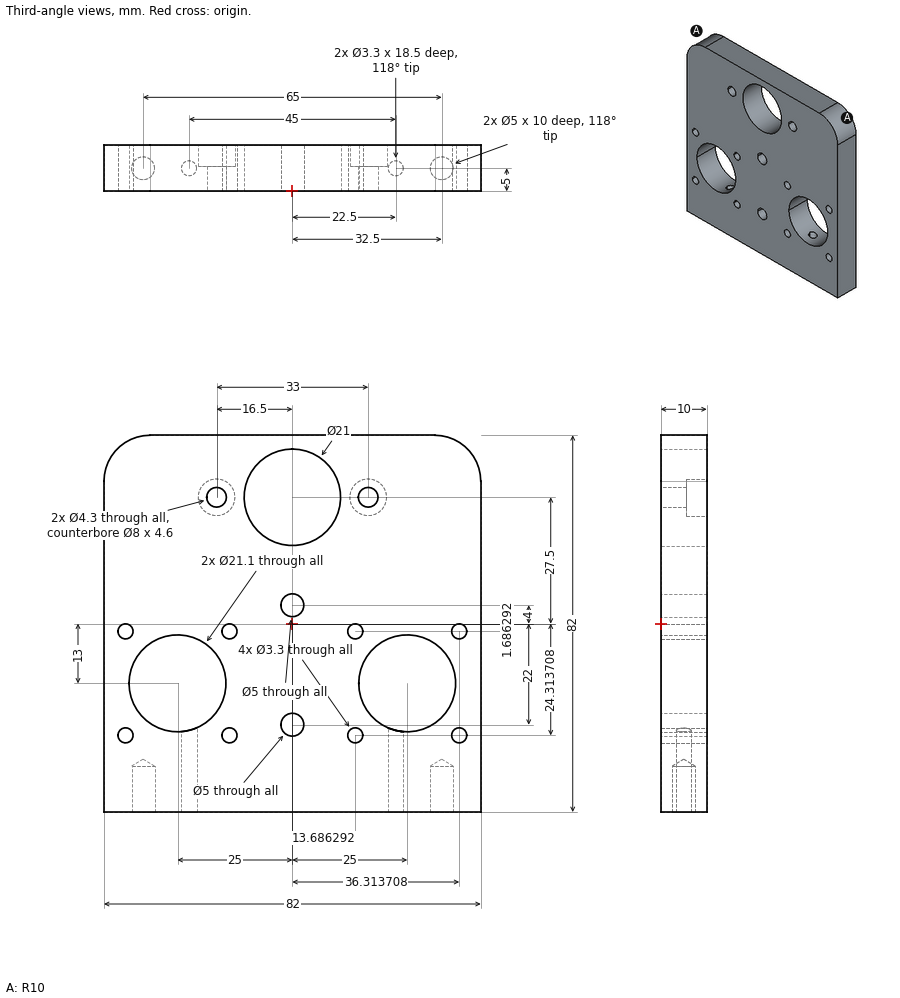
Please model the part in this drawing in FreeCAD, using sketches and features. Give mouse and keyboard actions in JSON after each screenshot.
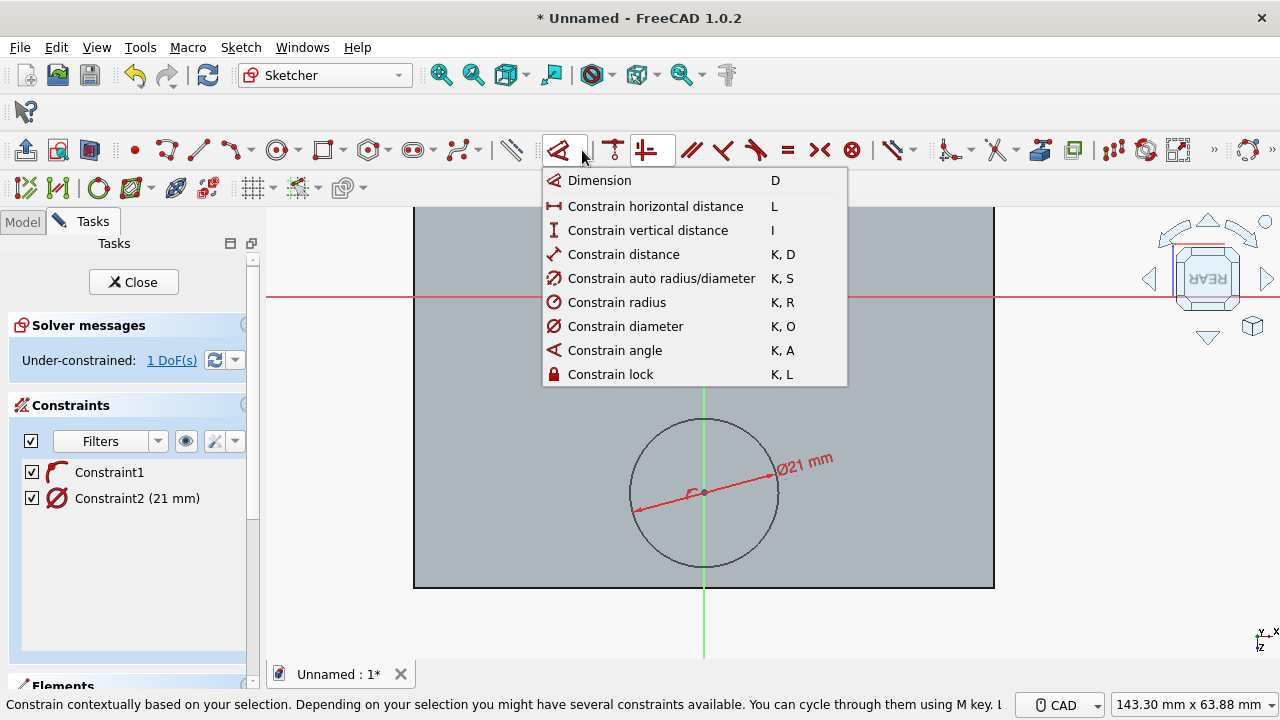
{"action": "left_click", "coordinate": [695, 230]}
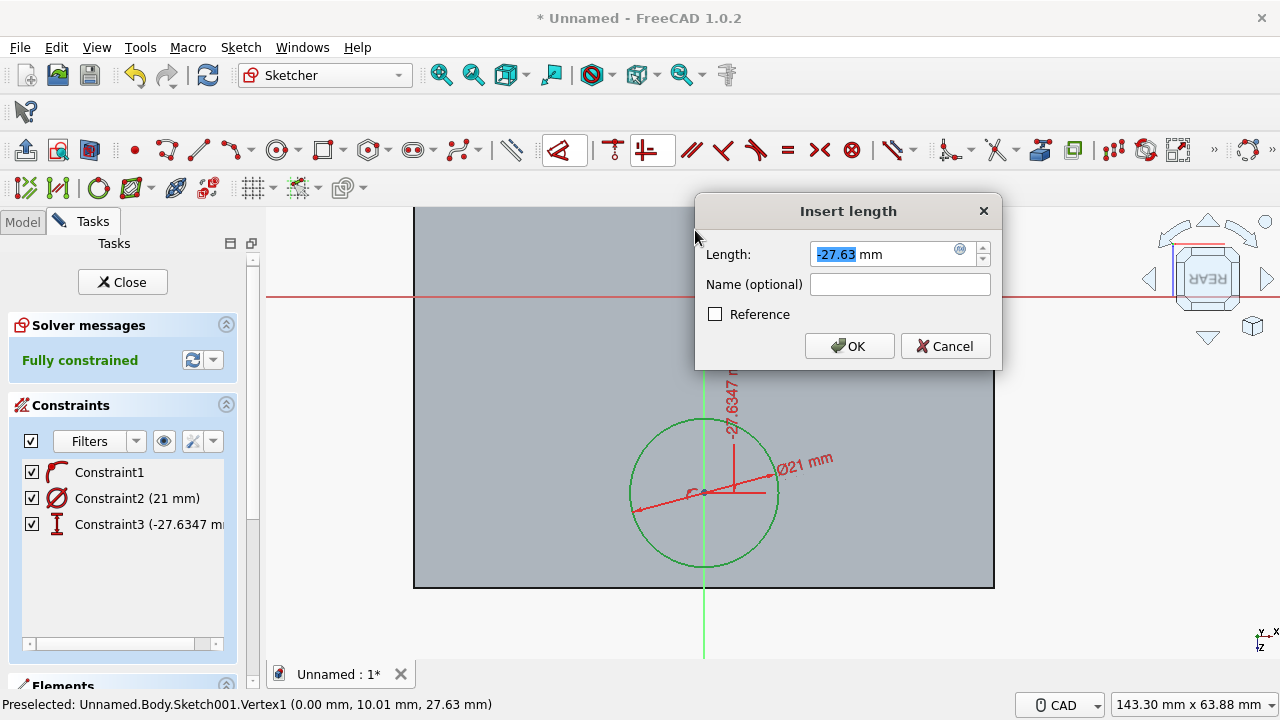
{"action": "type", "text": "-27.5"}
{"action": "key", "text": "Return"}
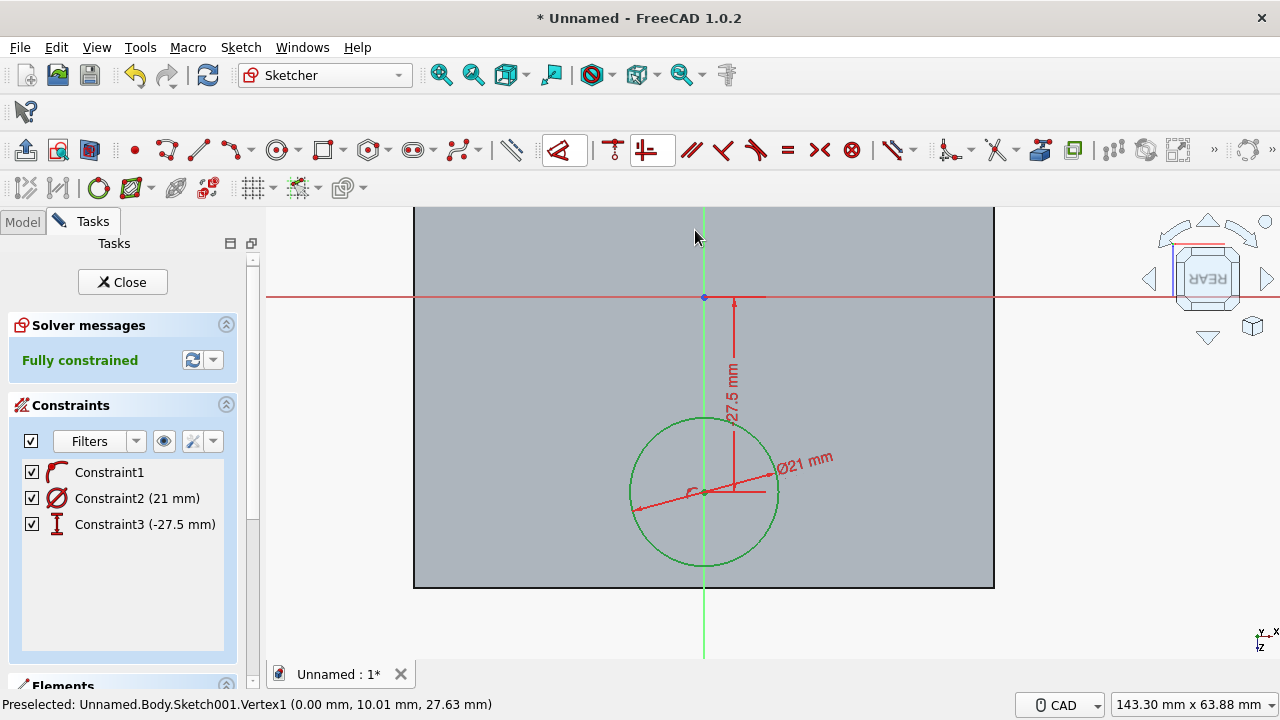
{"action": "left_click", "coordinate": [123, 282]}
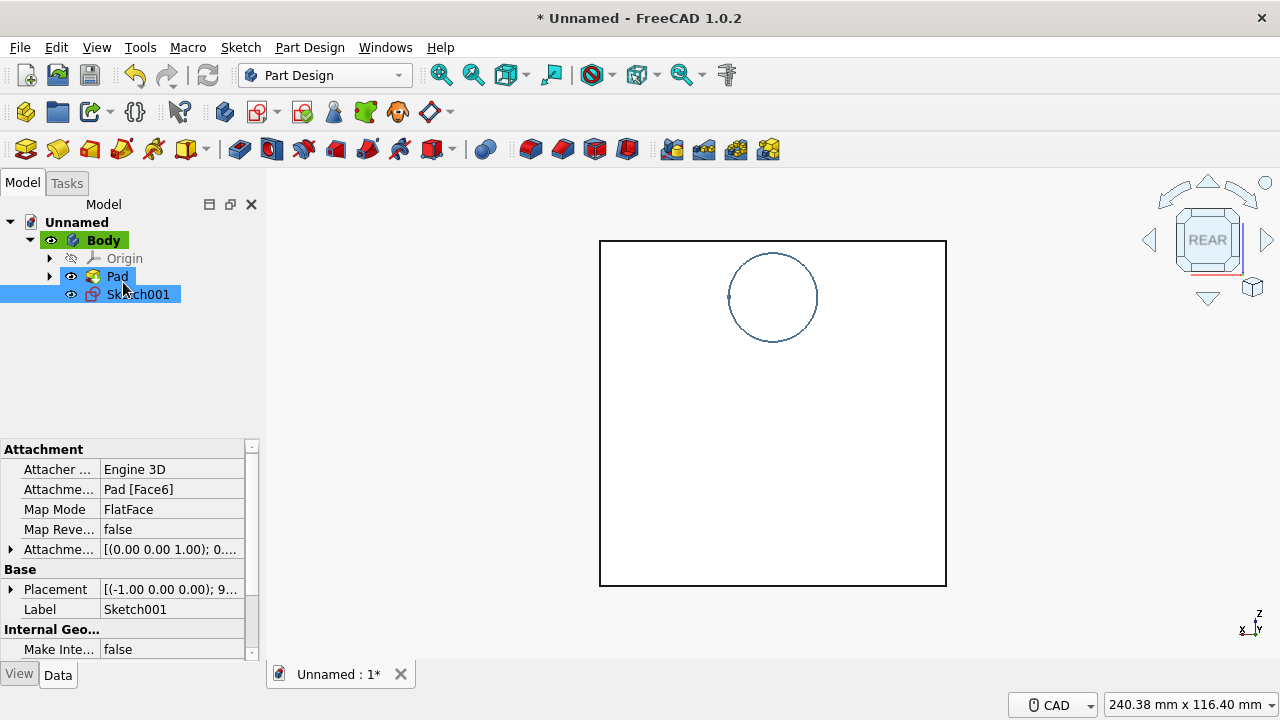
{"action": "left_click", "coordinate": [240, 150]}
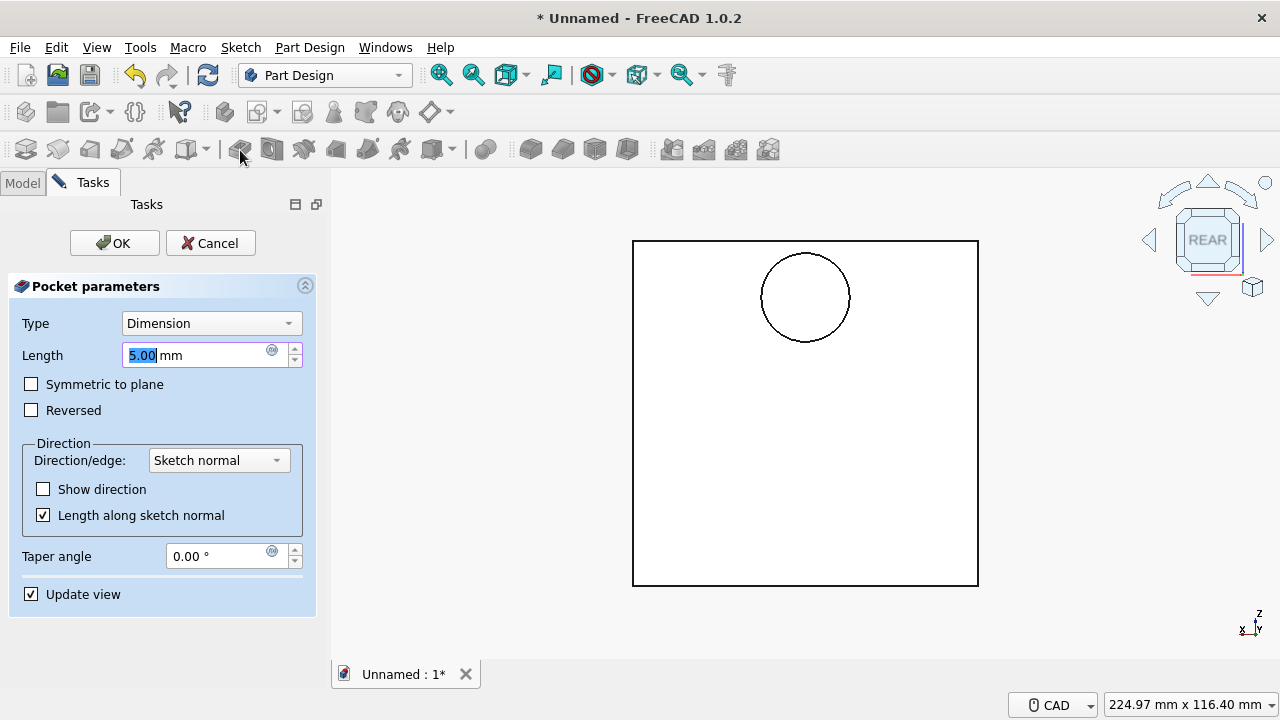
{"action": "left_click", "coordinate": [212, 324]}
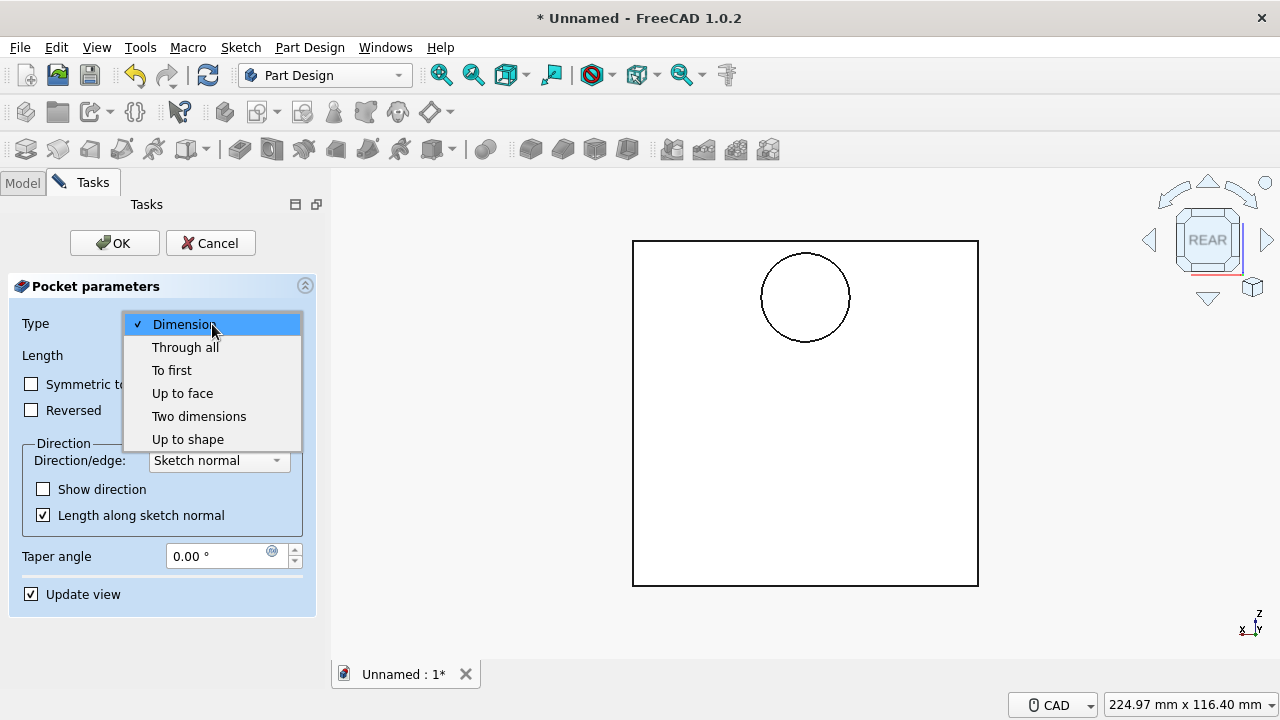
{"action": "left_click", "coordinate": [212, 348]}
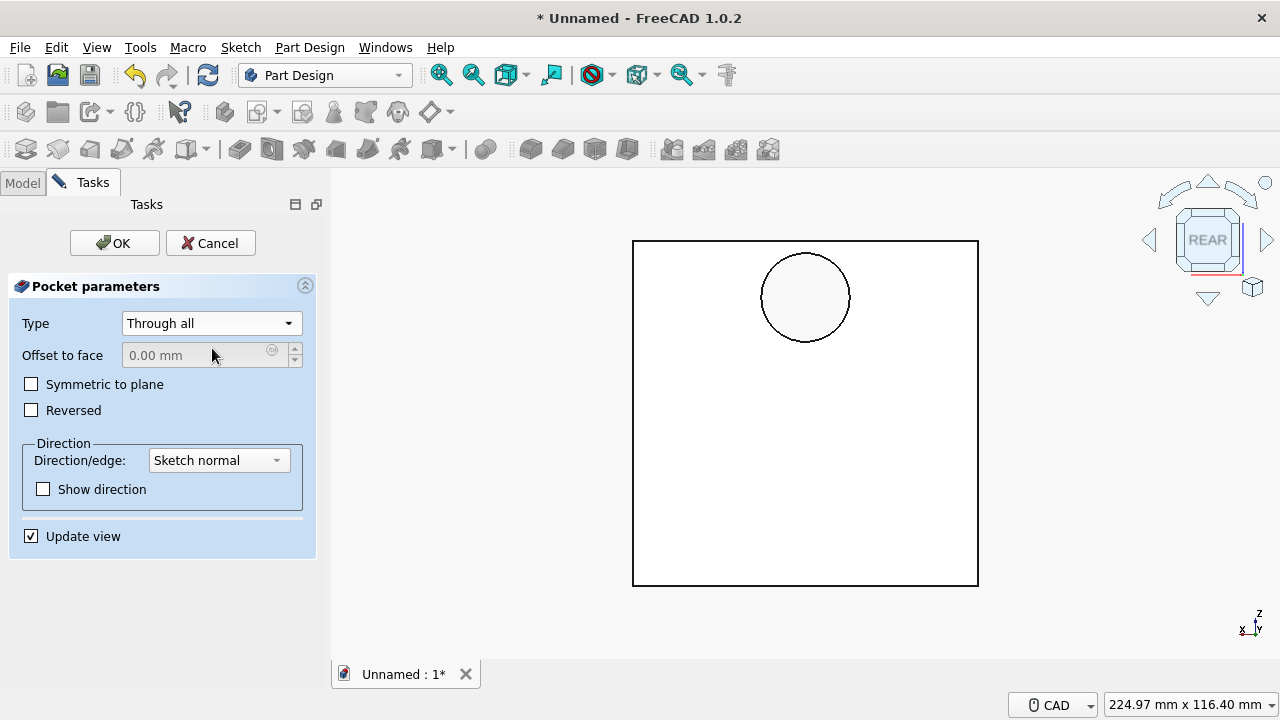
{"action": "left_click", "coordinate": [115, 243]}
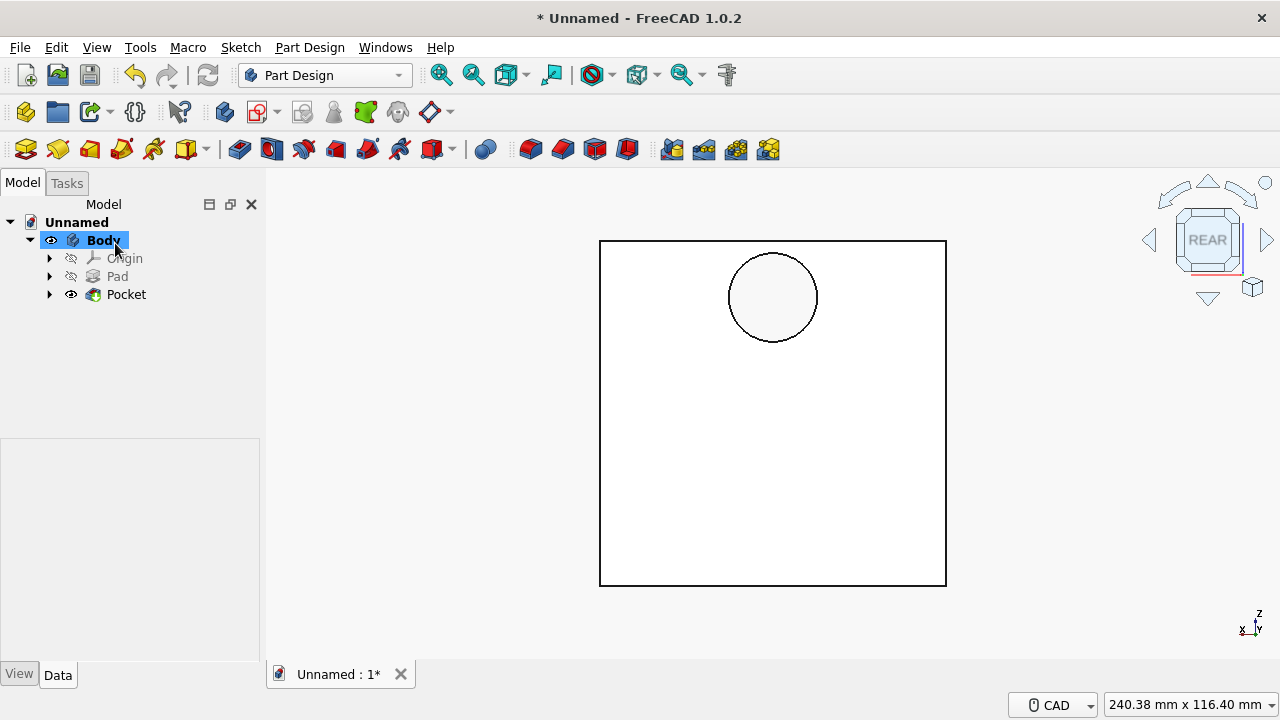
{"action": "key", "text": "0"}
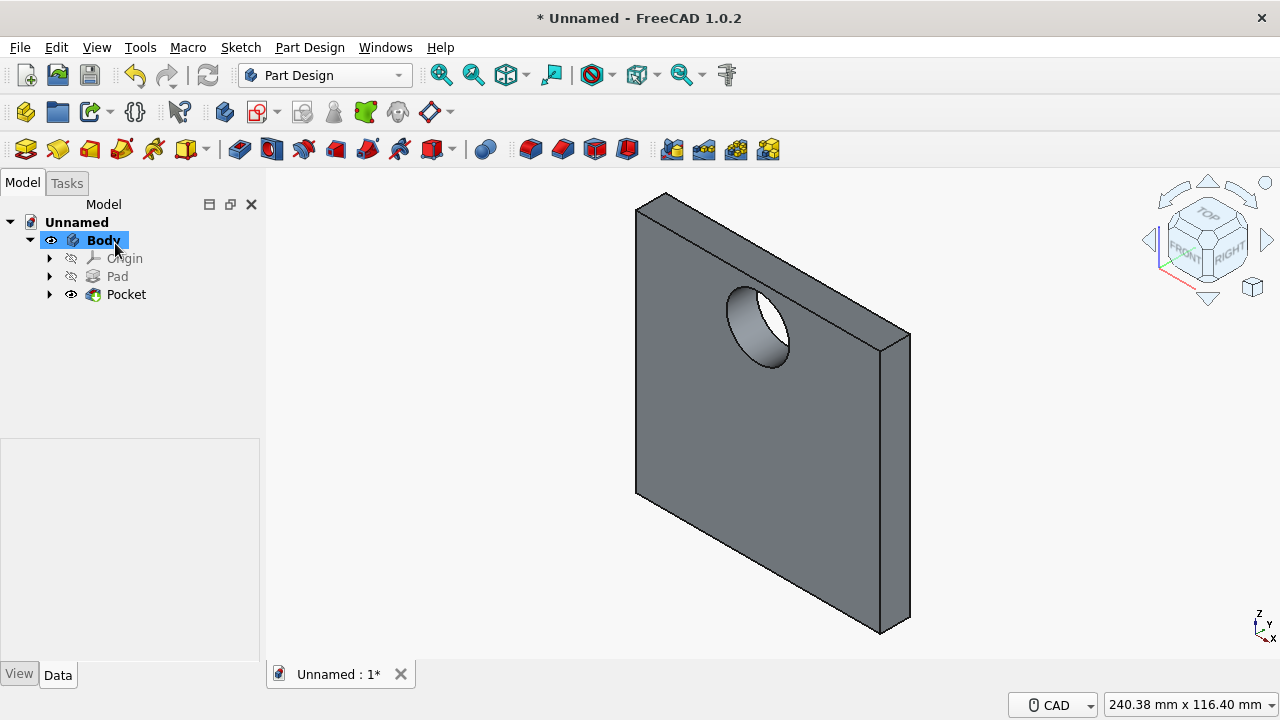
{"action": "left_click", "coordinate": [895, 342]}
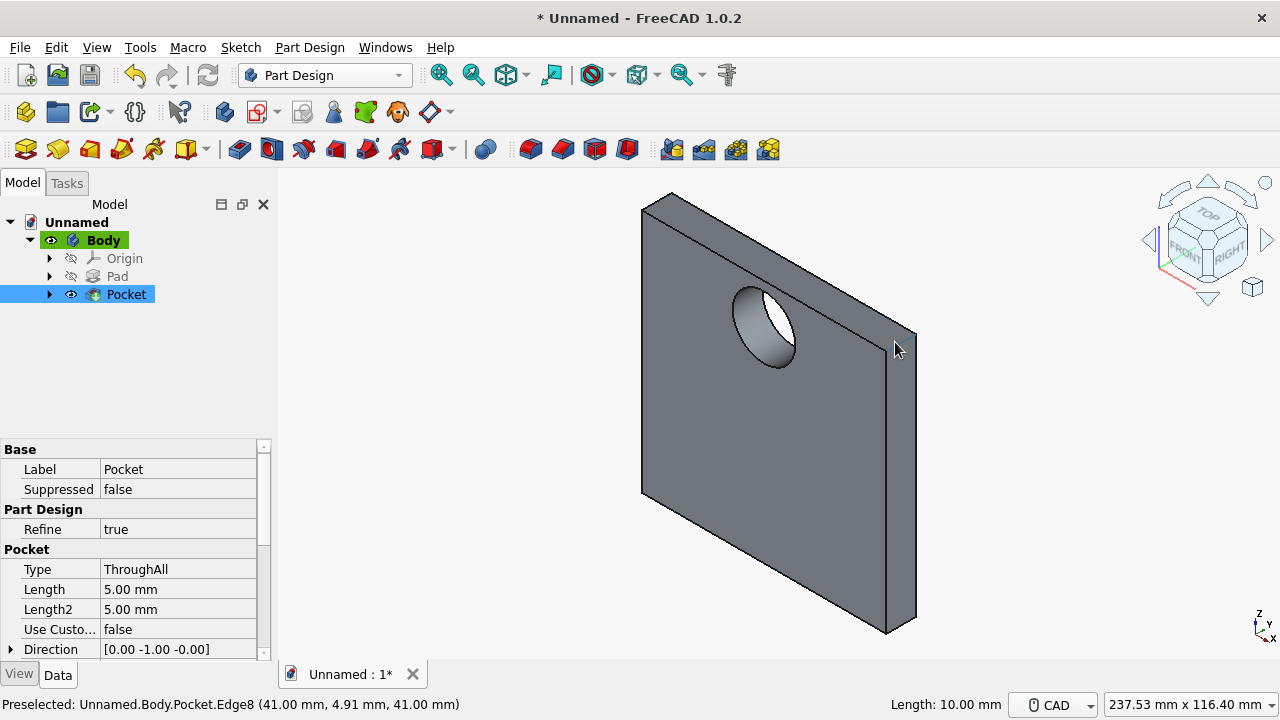
{"action": "key", "text": "2"}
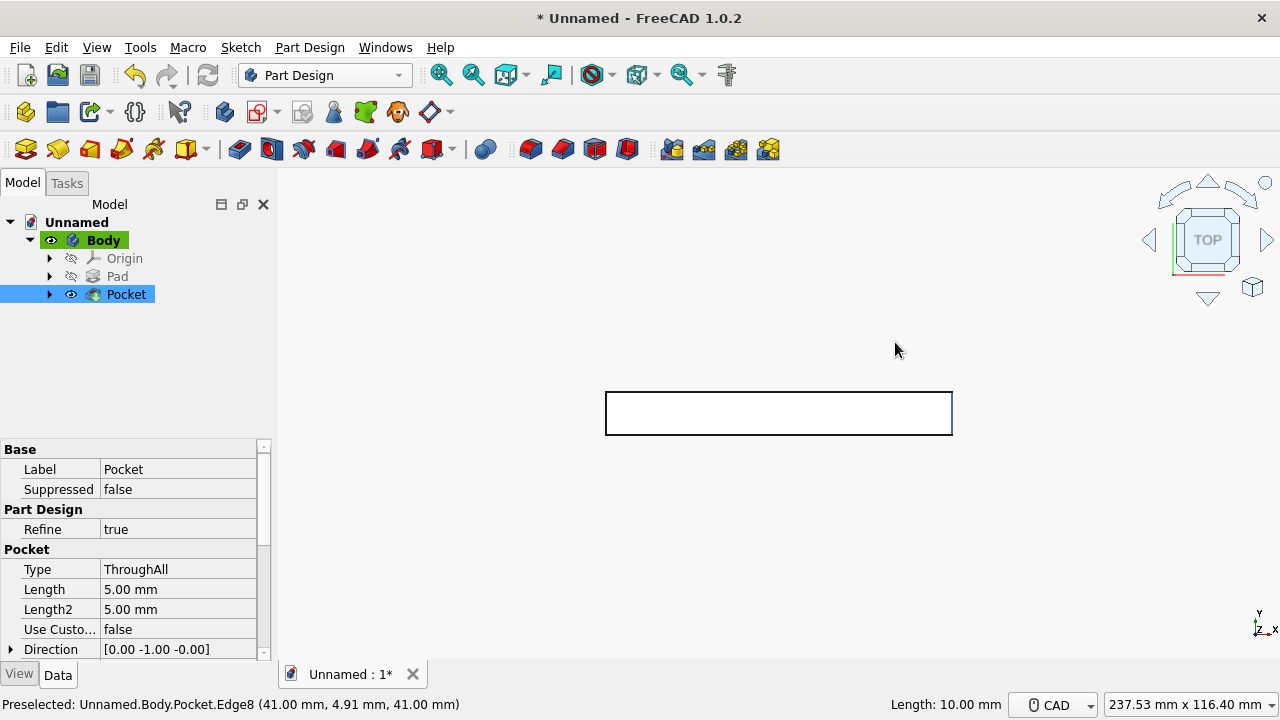
{"action": "left_click", "coordinate": [442, 76]}